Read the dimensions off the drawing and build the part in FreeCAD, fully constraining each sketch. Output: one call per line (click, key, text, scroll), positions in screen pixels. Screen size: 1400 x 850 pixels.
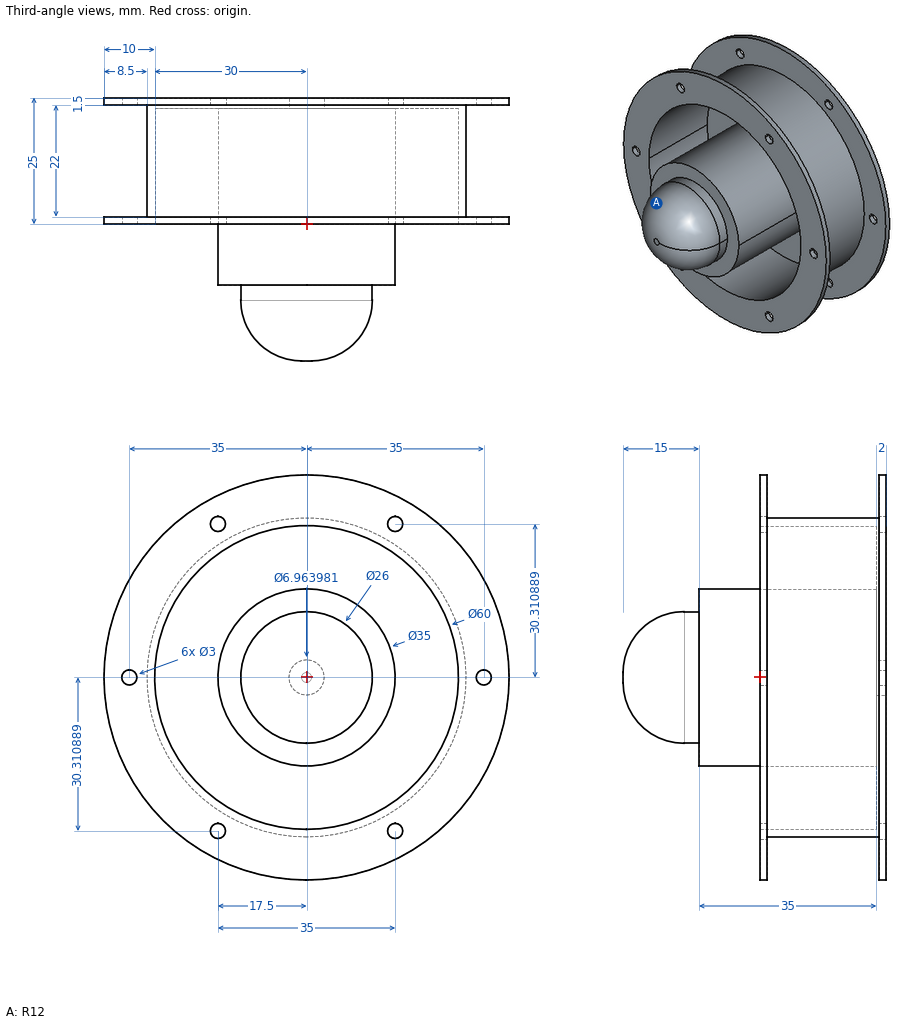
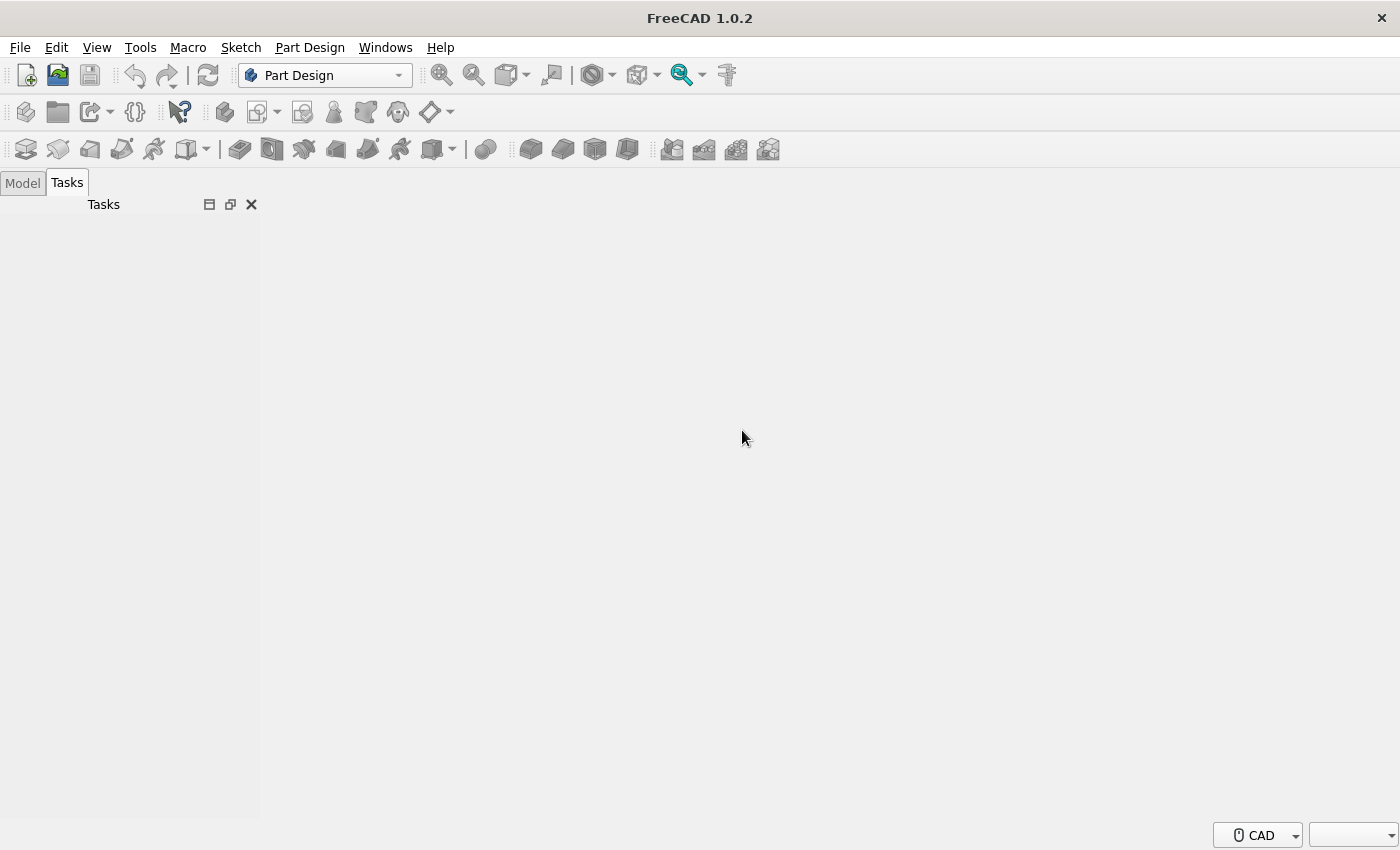
click(26, 76)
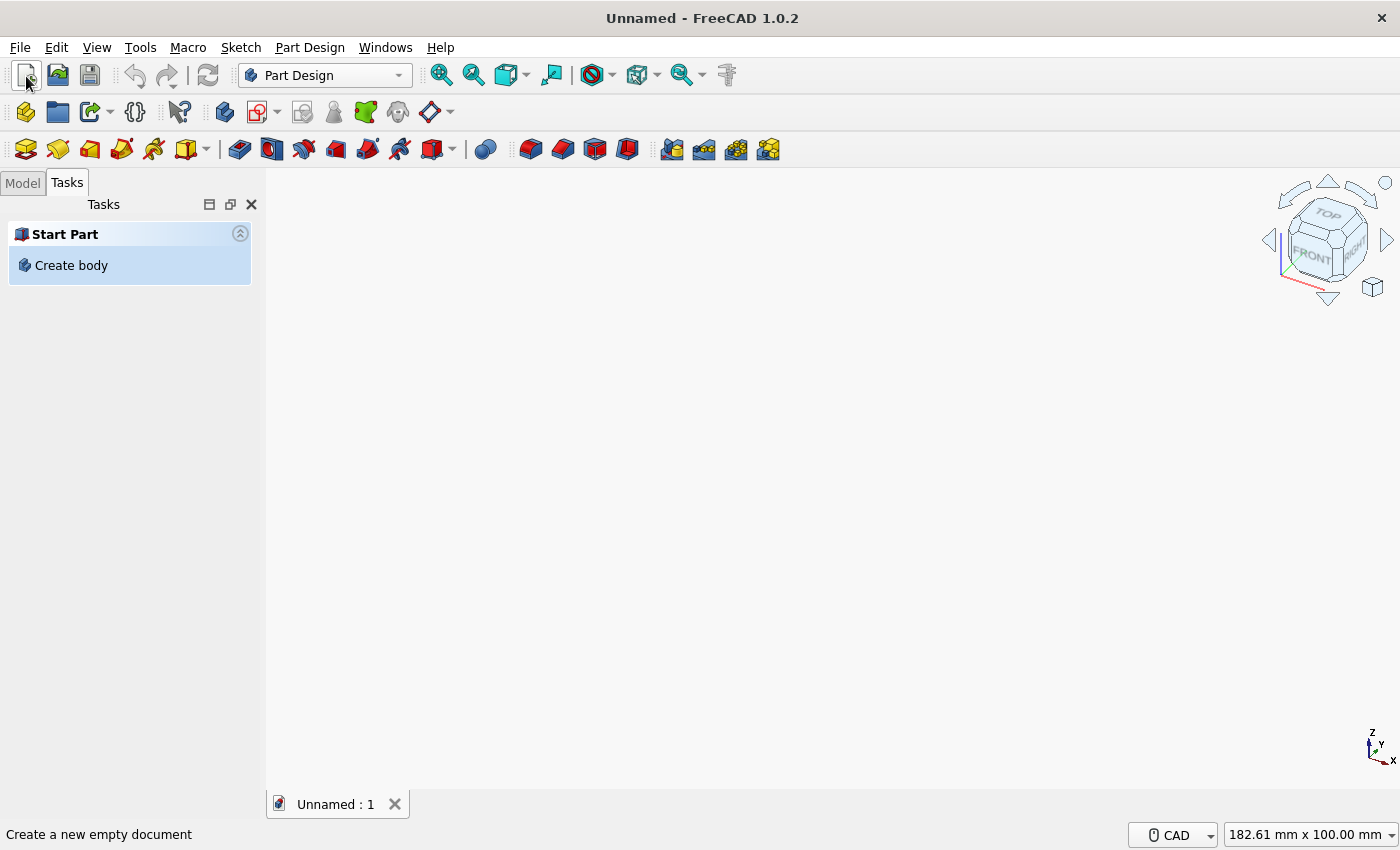
click(258, 112)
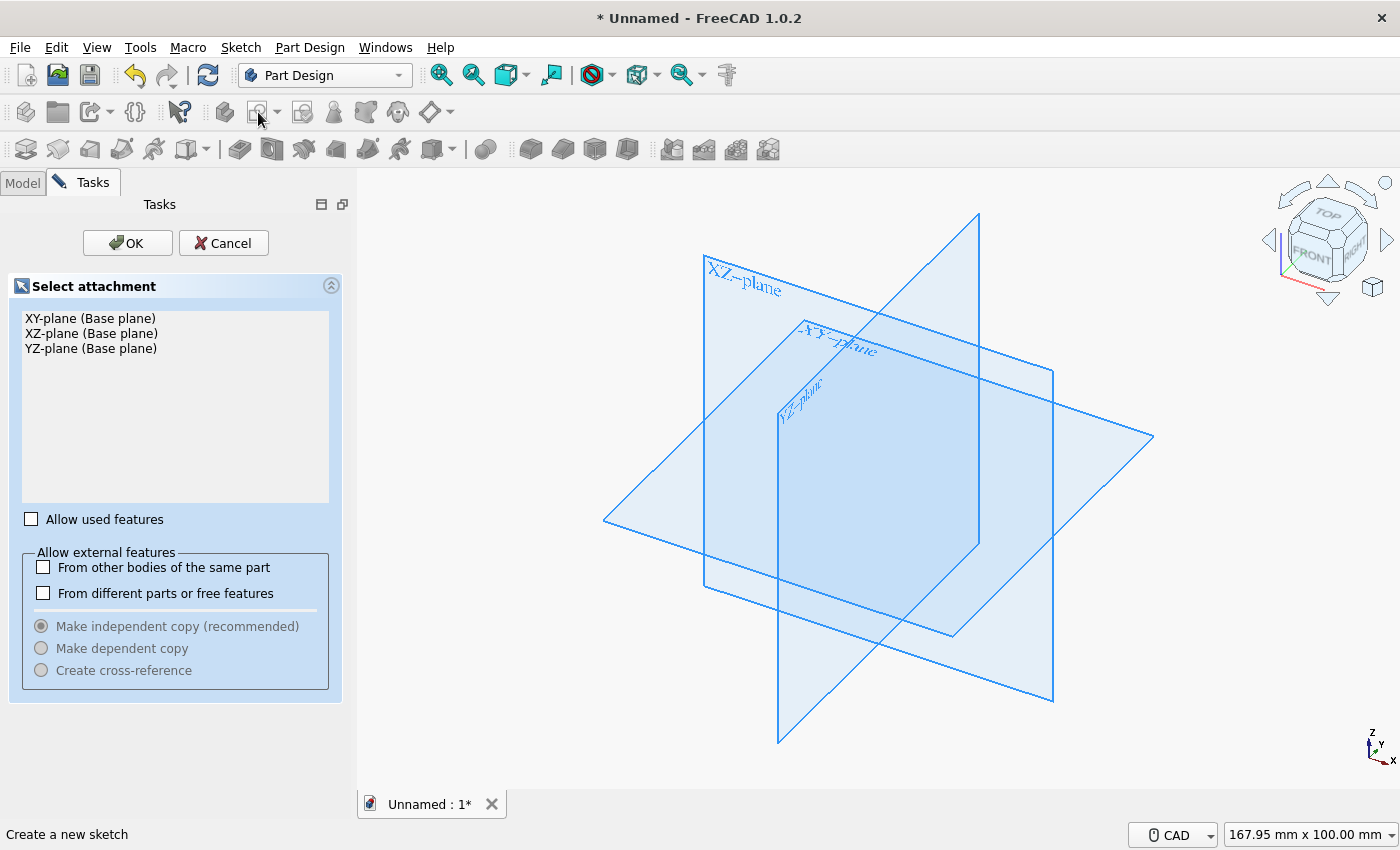
click(82, 318)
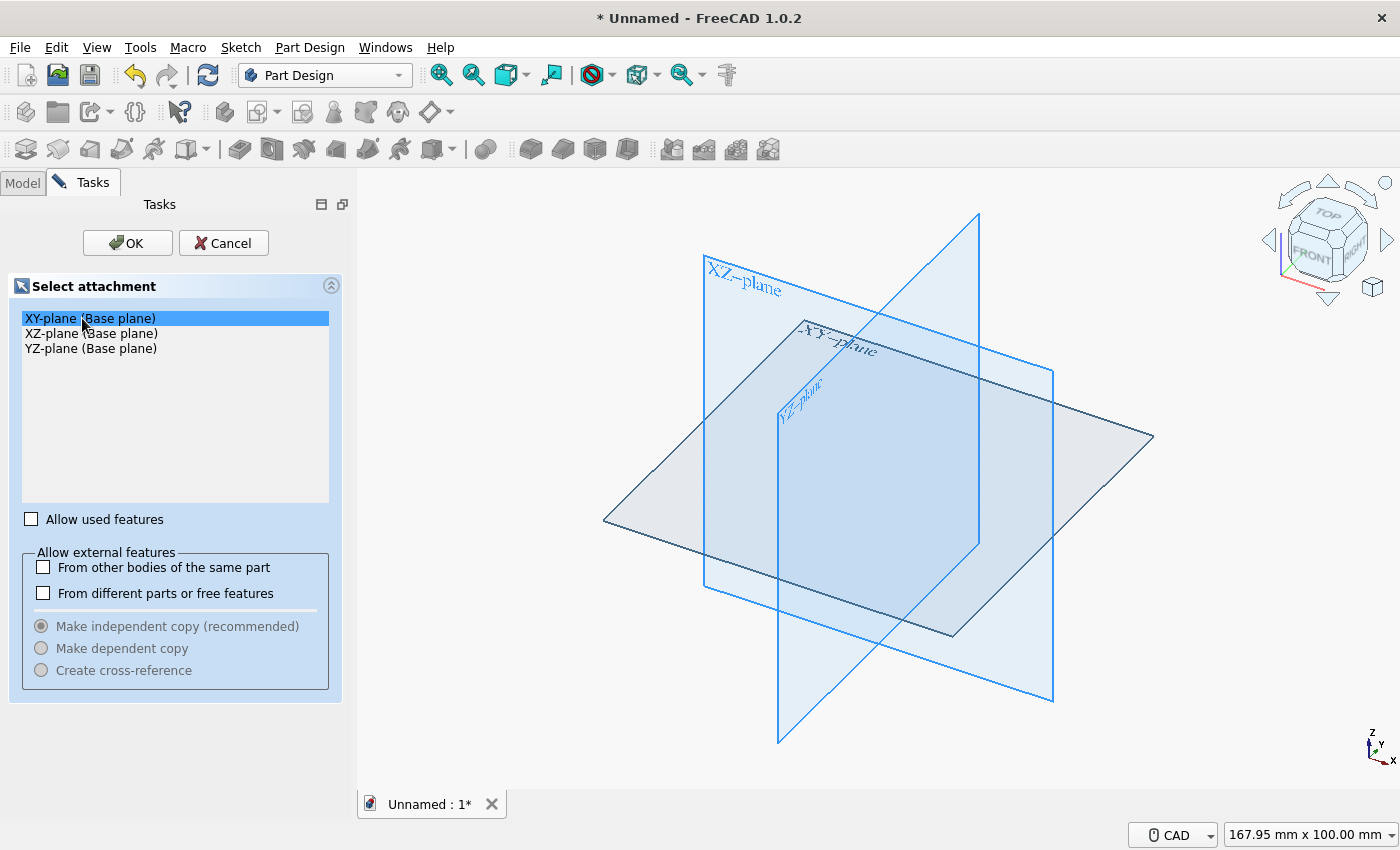
click(128, 243)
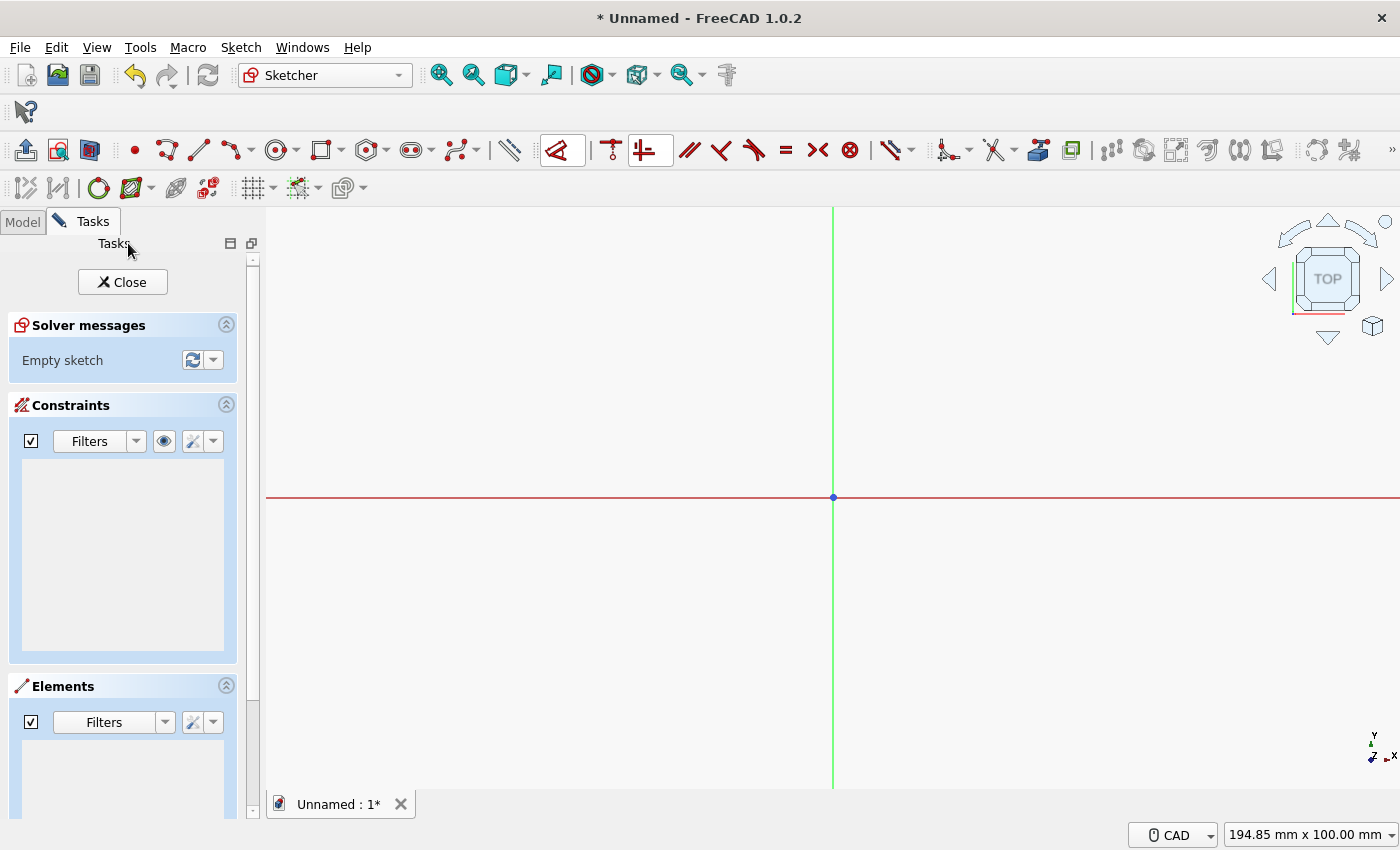
scroll(689, 383, up, 5)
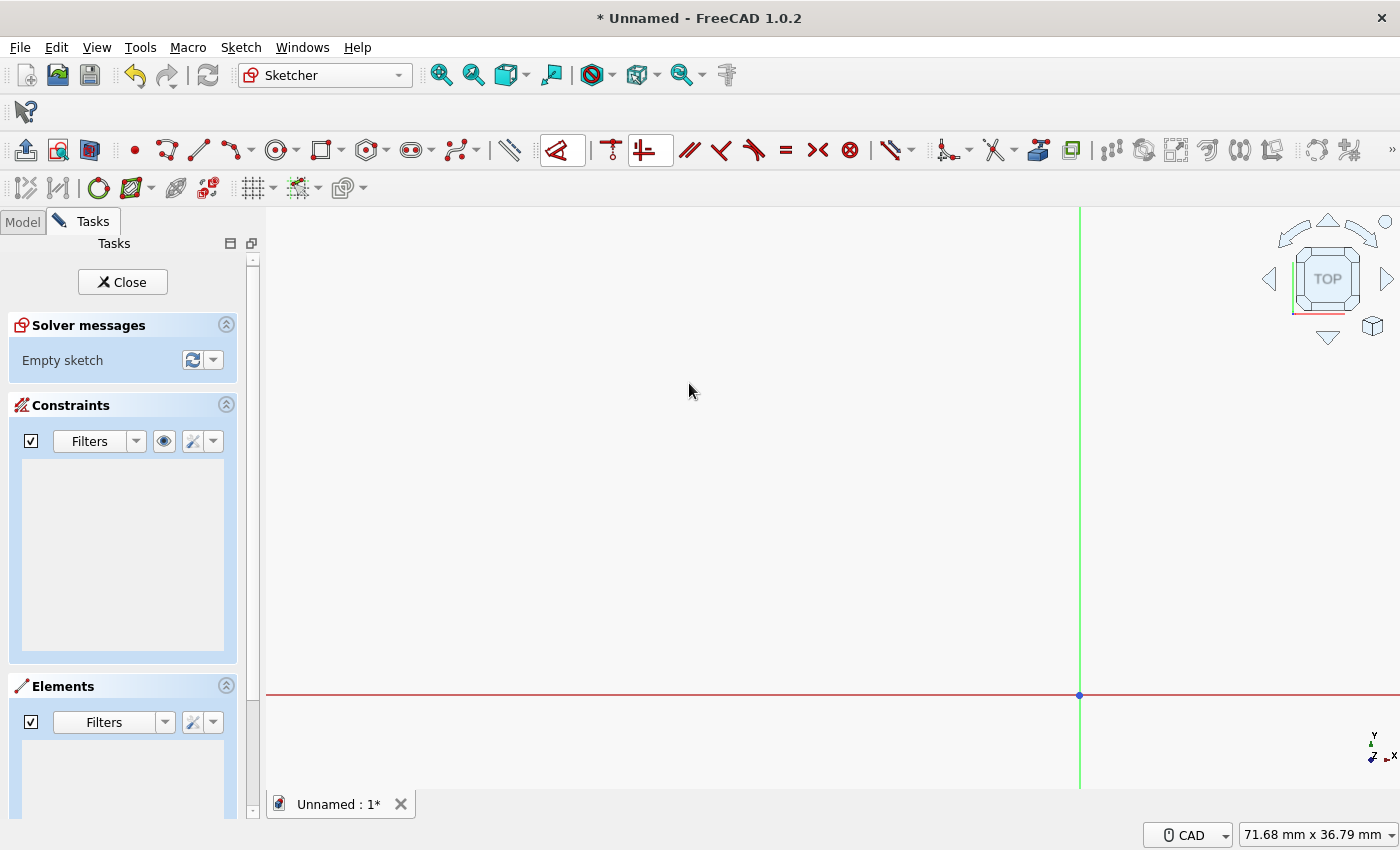
click(168, 150)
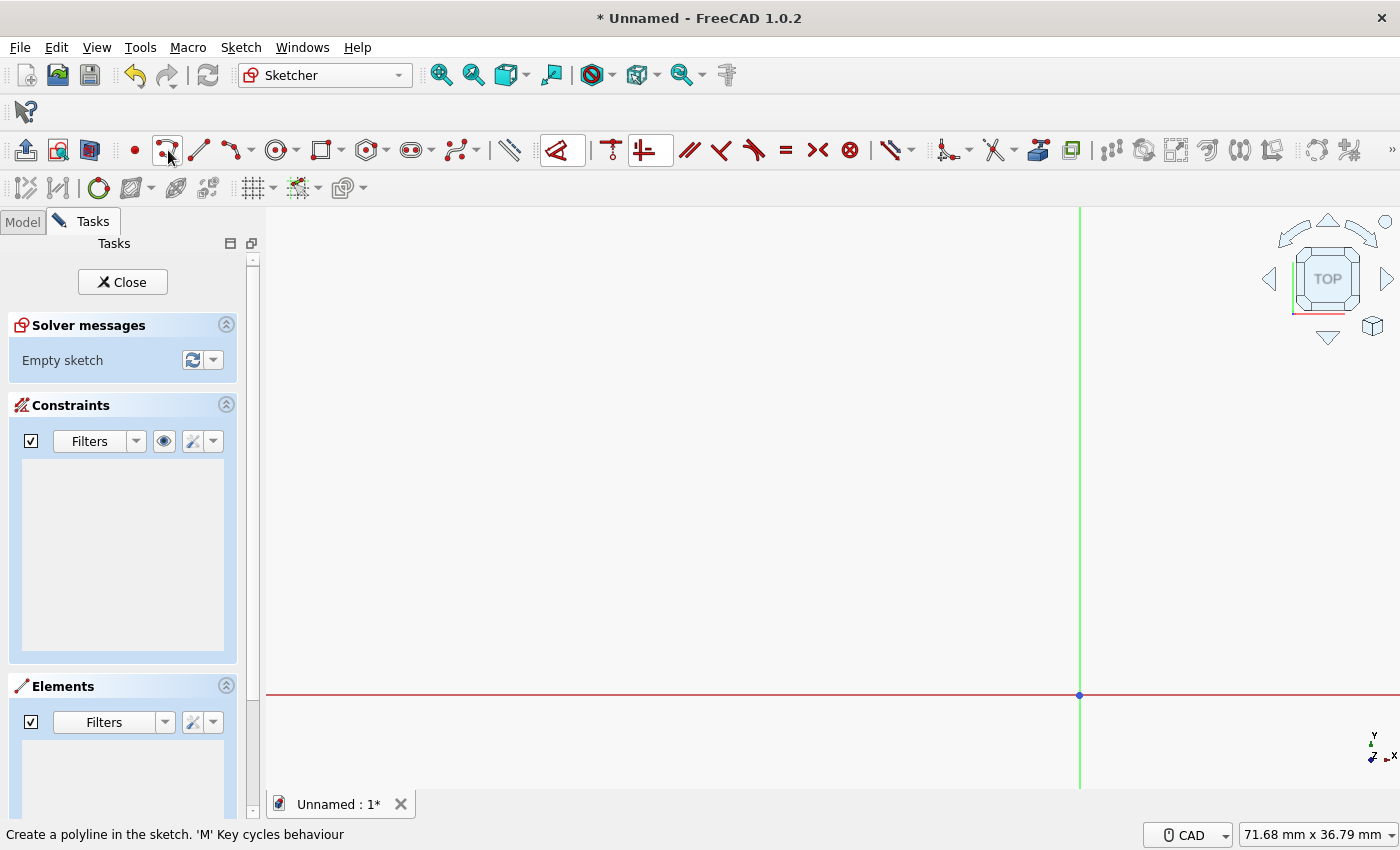
click(605, 695)
click(605, 300)
click(447, 300)
click(447, 323)
click(581, 323)
click(581, 671)
click(447, 671)
click(447, 686)
click(605, 695)
key(Escape)
key(Escape)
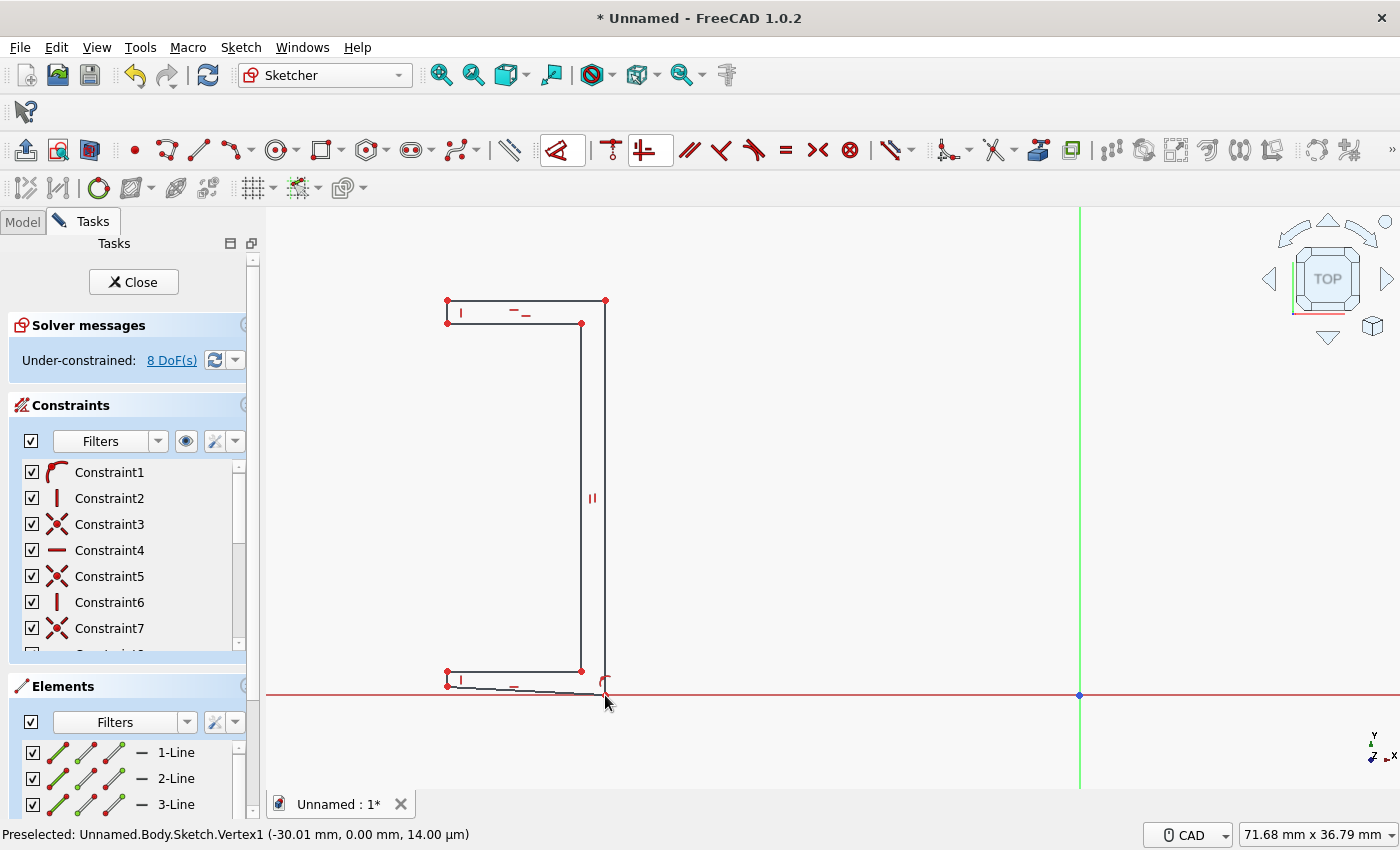
click(558, 693)